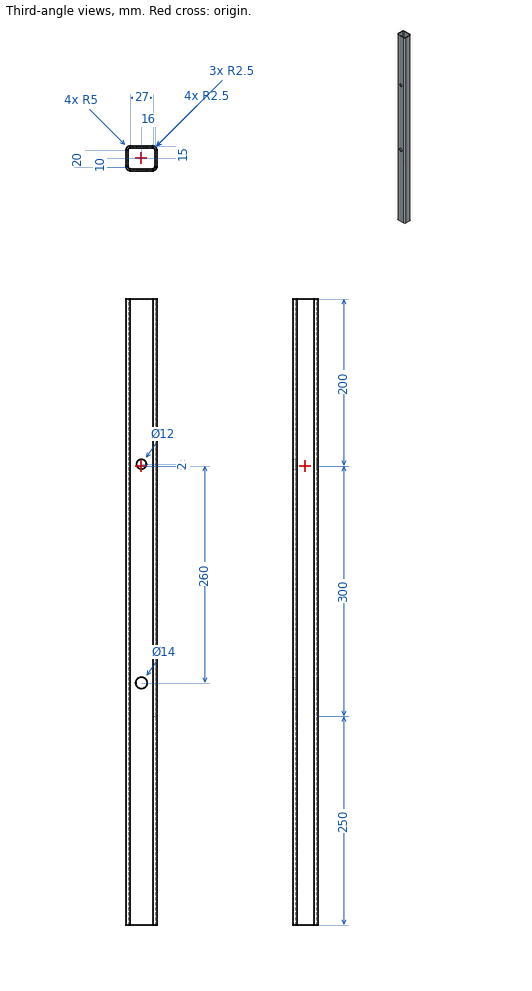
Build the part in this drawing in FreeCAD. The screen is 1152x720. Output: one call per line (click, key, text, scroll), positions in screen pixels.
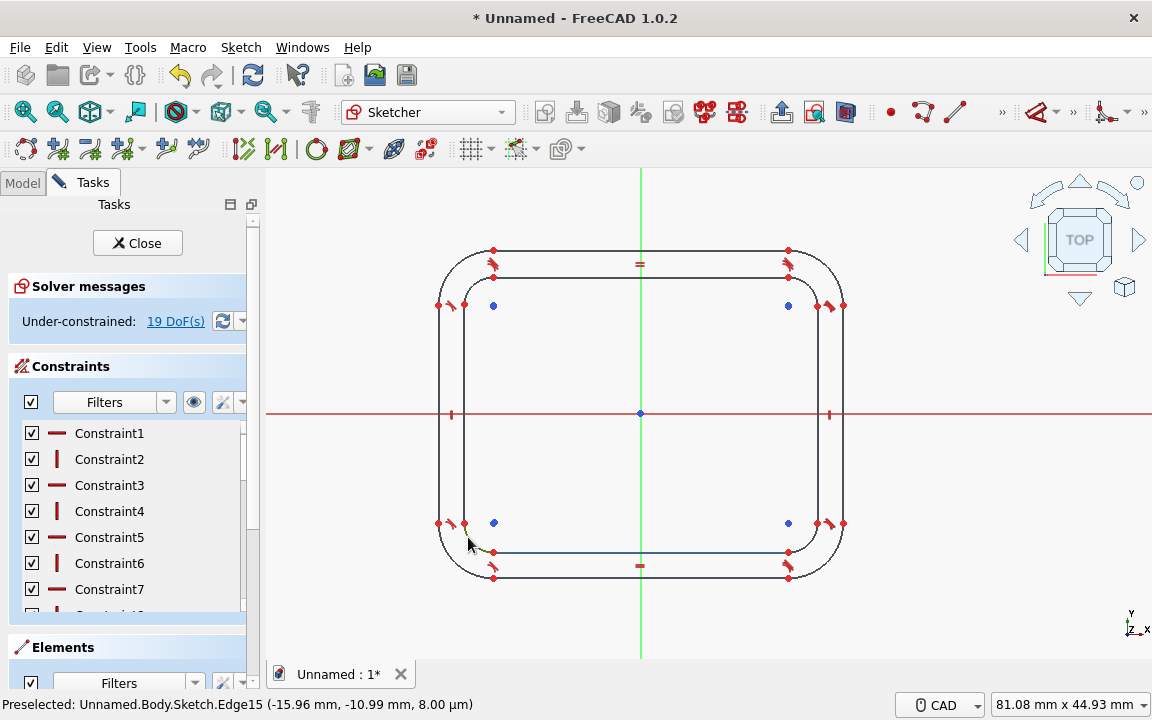
key(t)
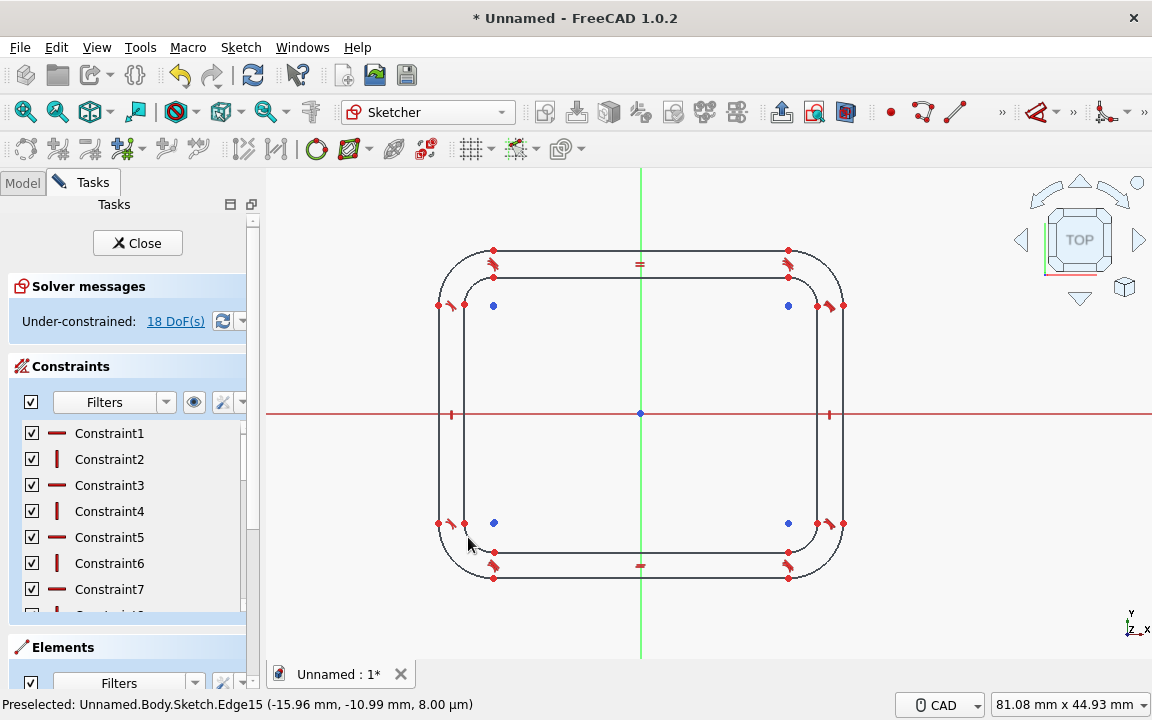
click(464, 458)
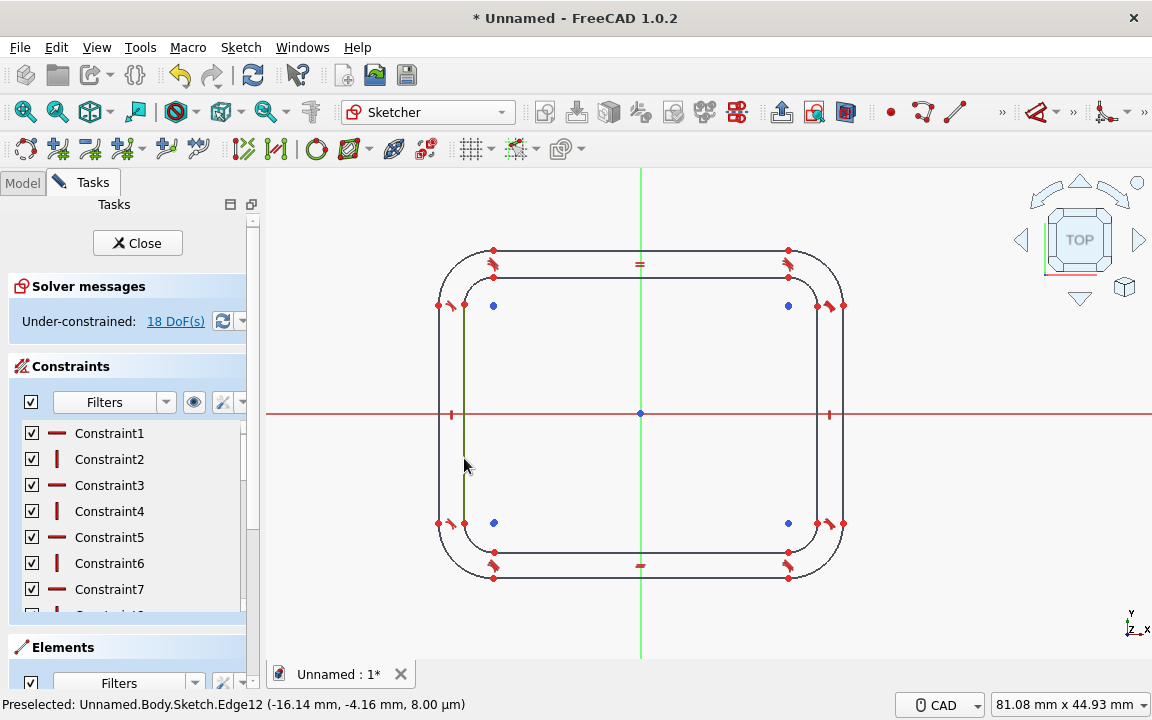
click(468, 537)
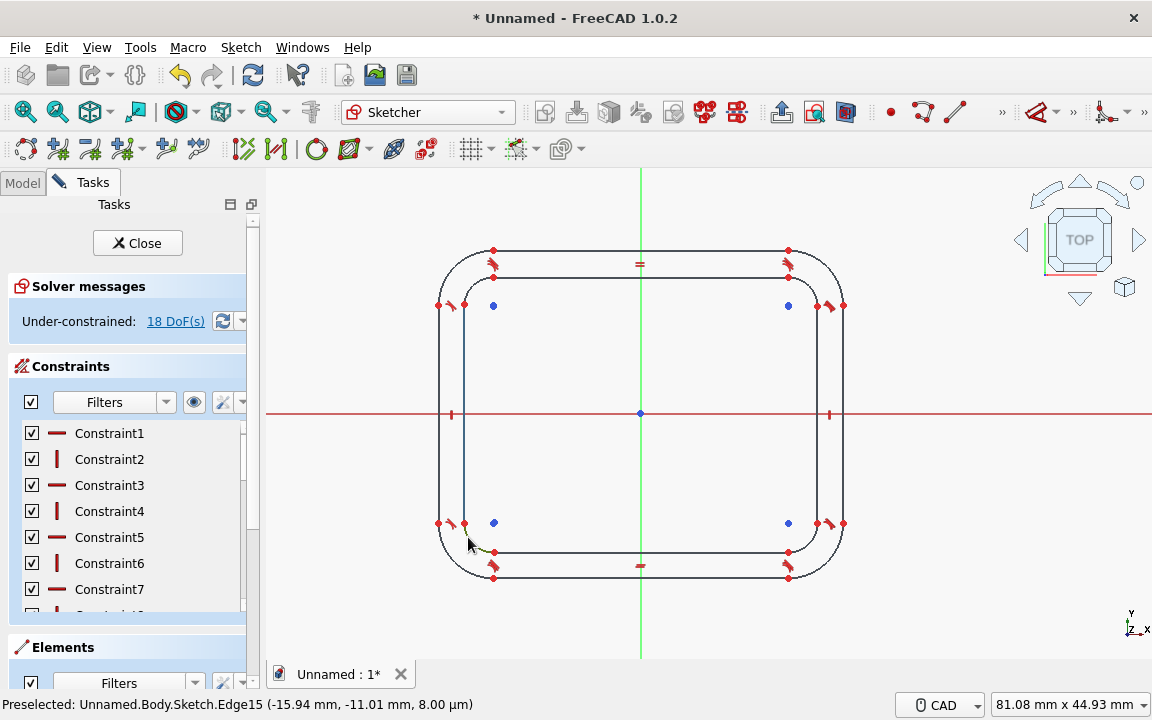
key(t)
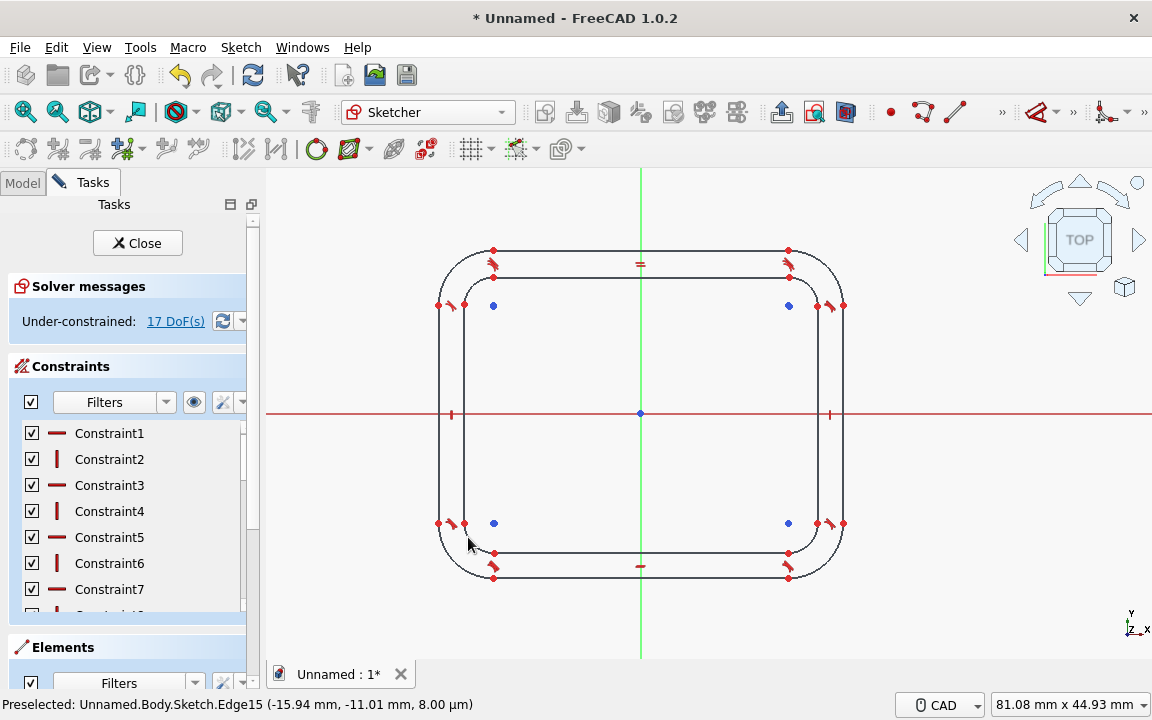
click(464, 458)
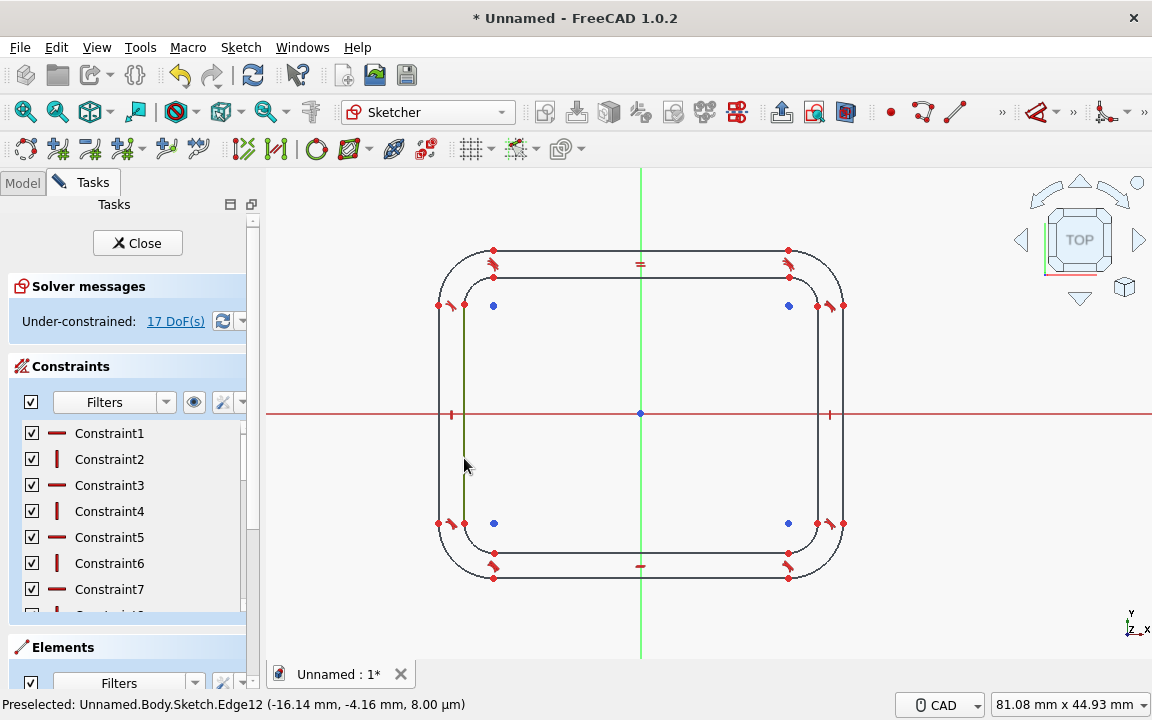
click(480, 281)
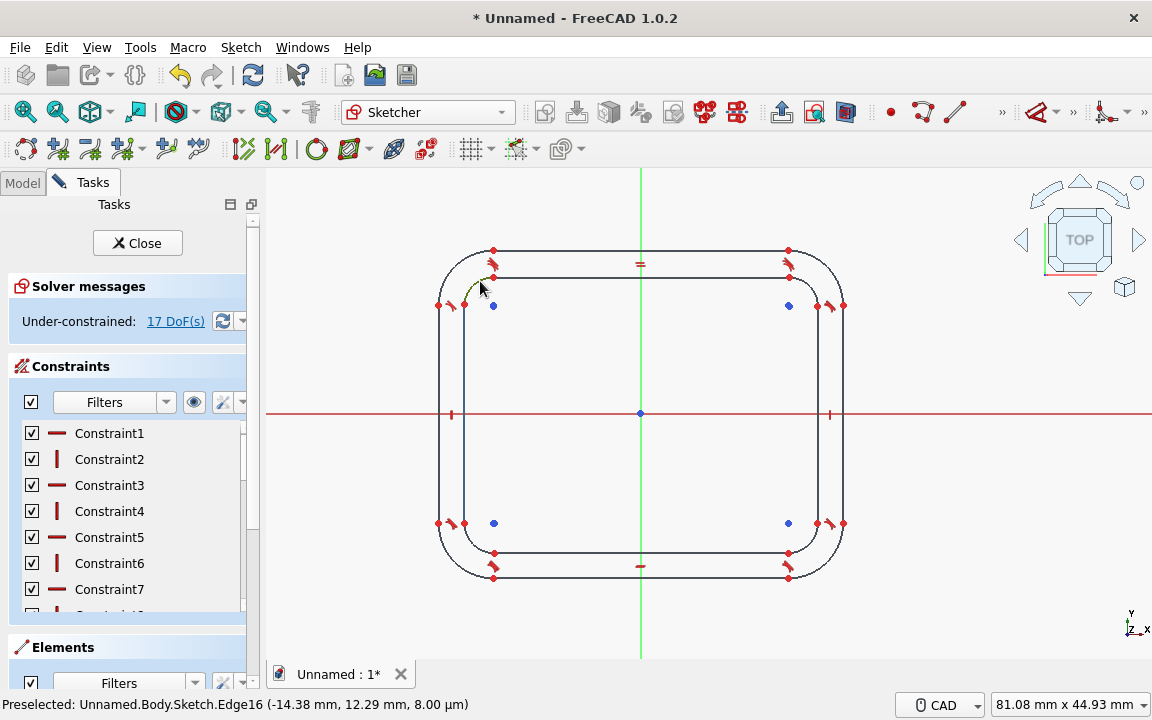
key(t)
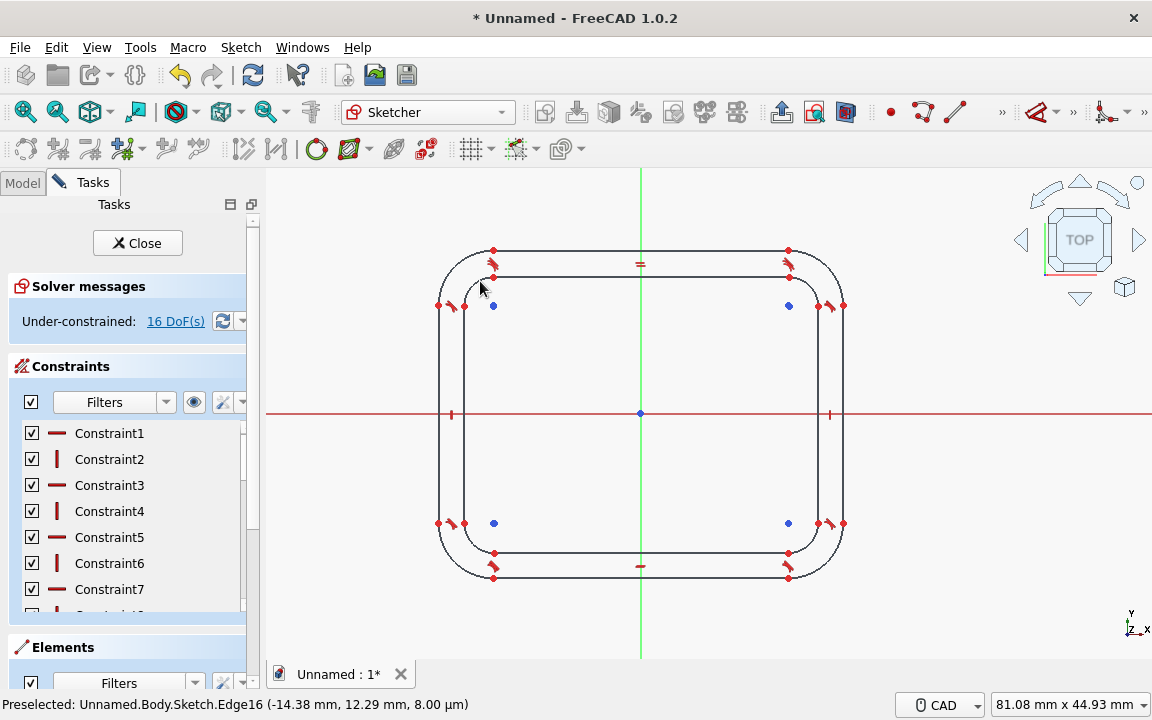
click(837, 281)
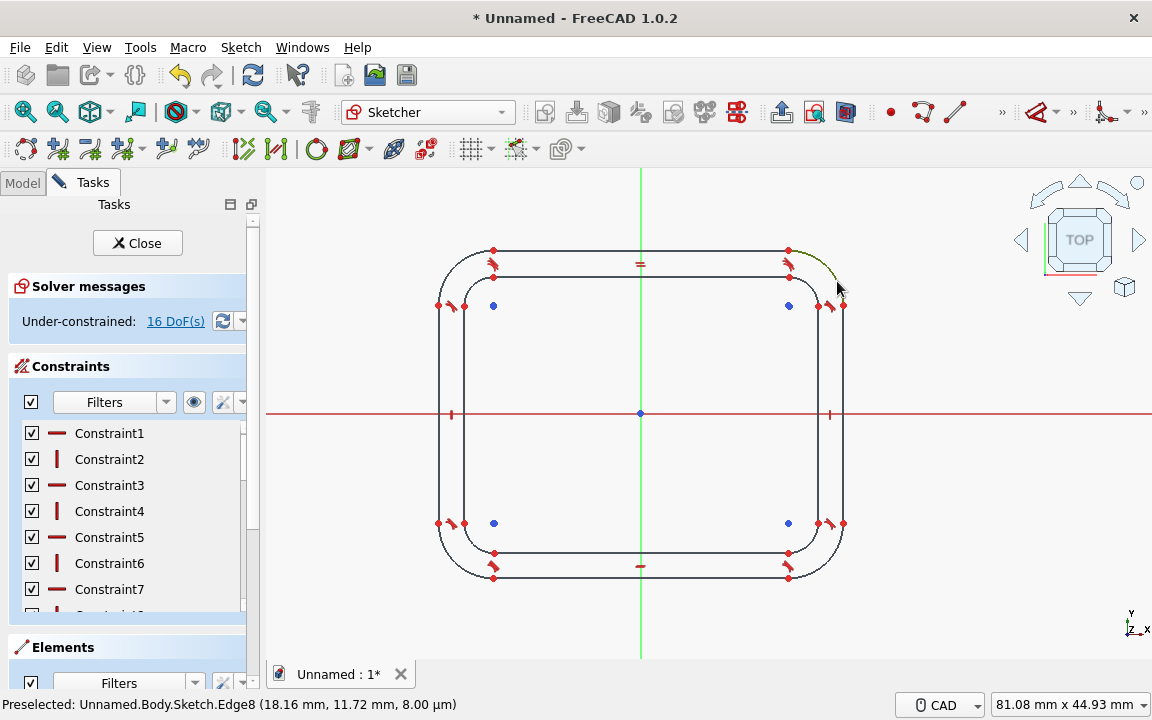
click(815, 293)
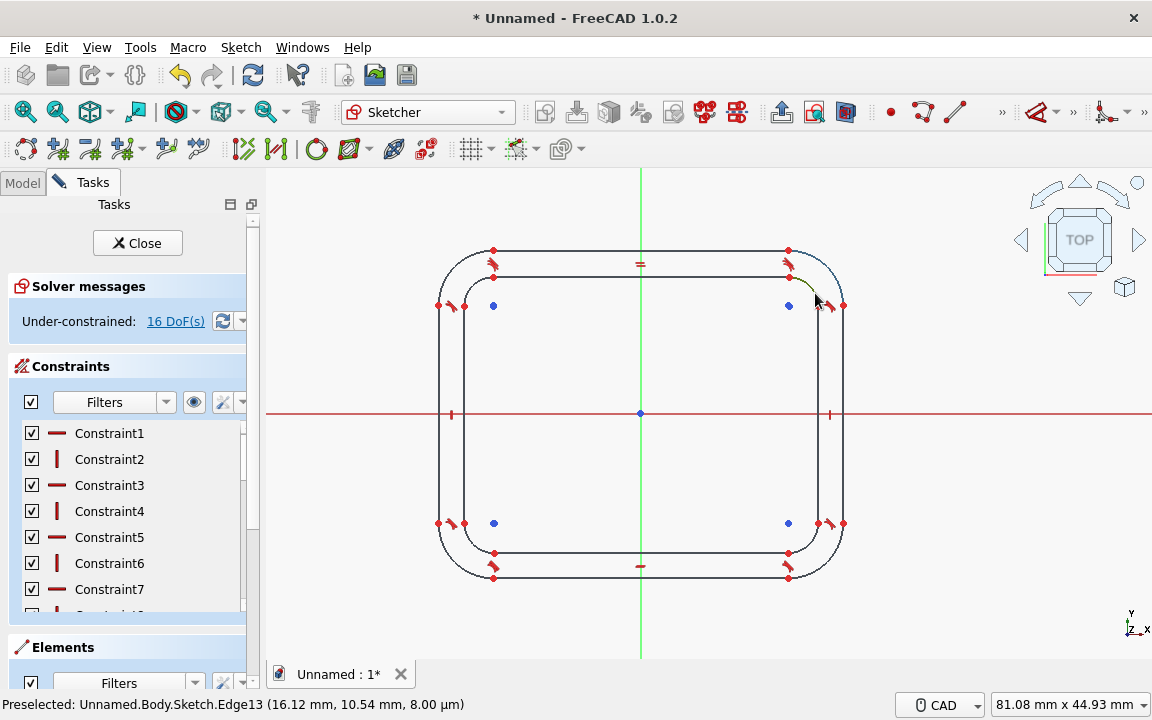
key(c)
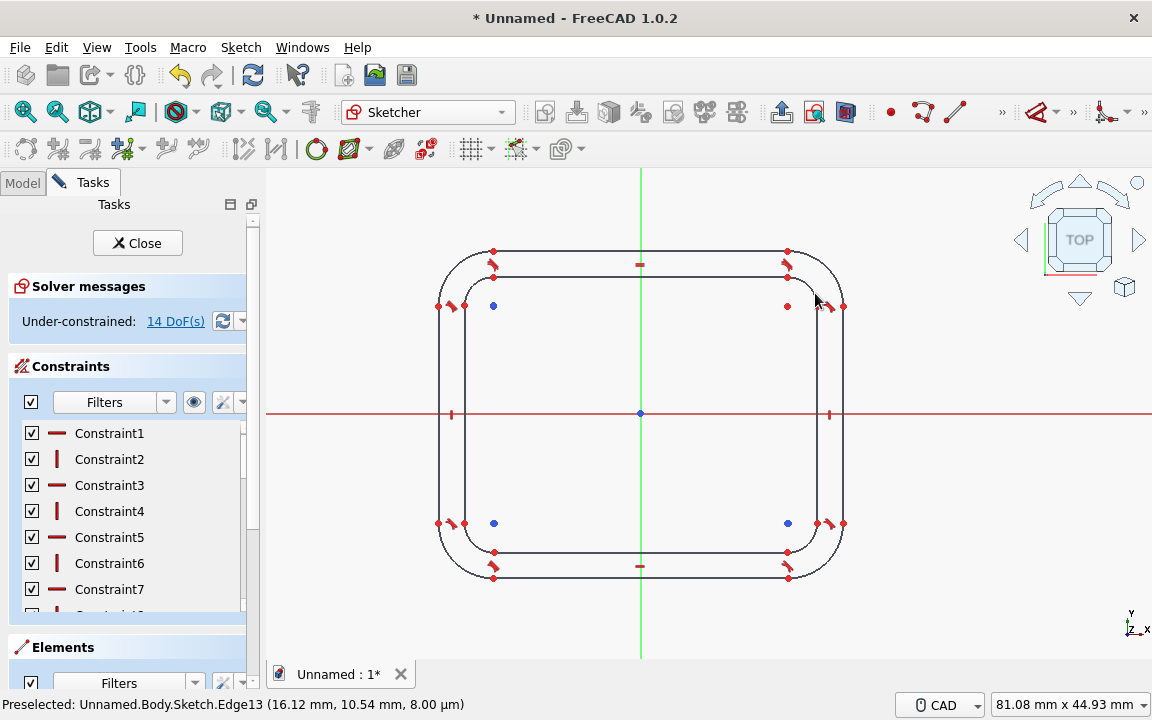
click(813, 572)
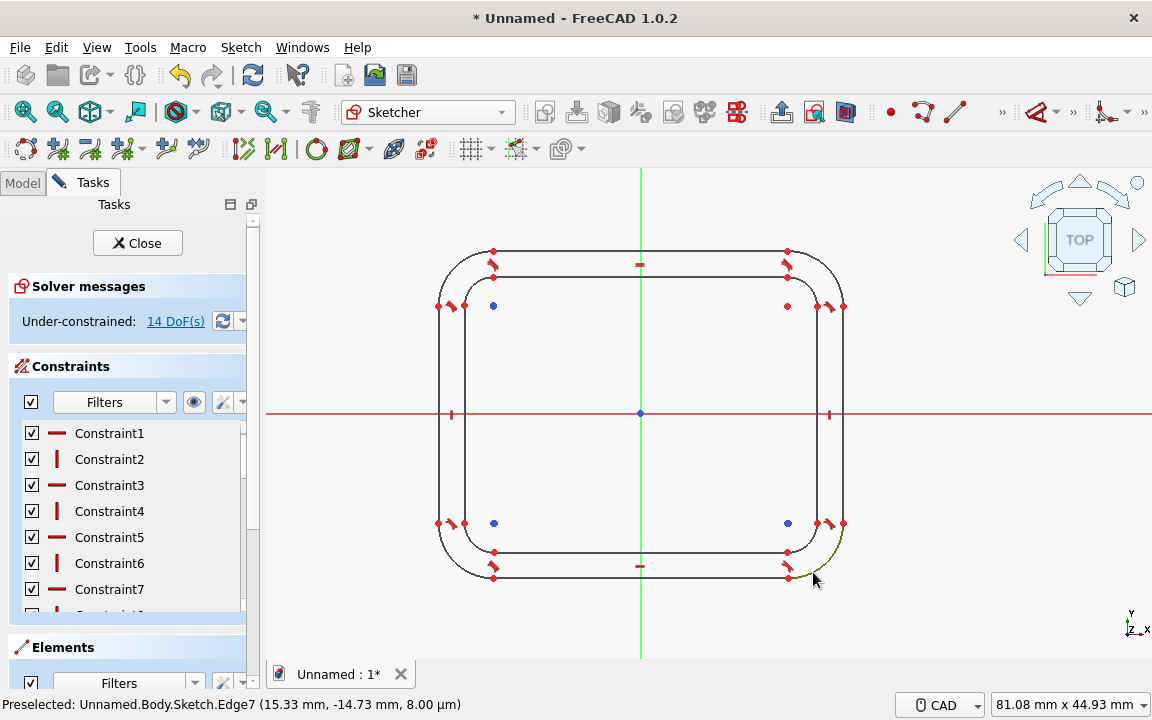
click(801, 550)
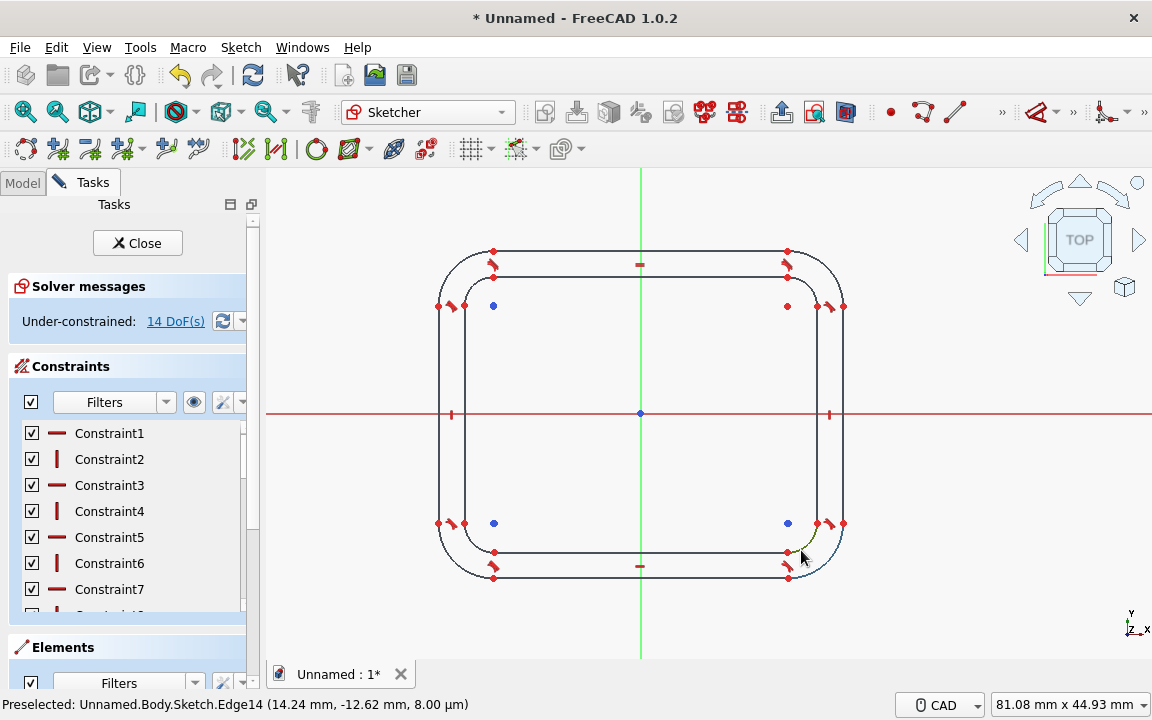
key(c)